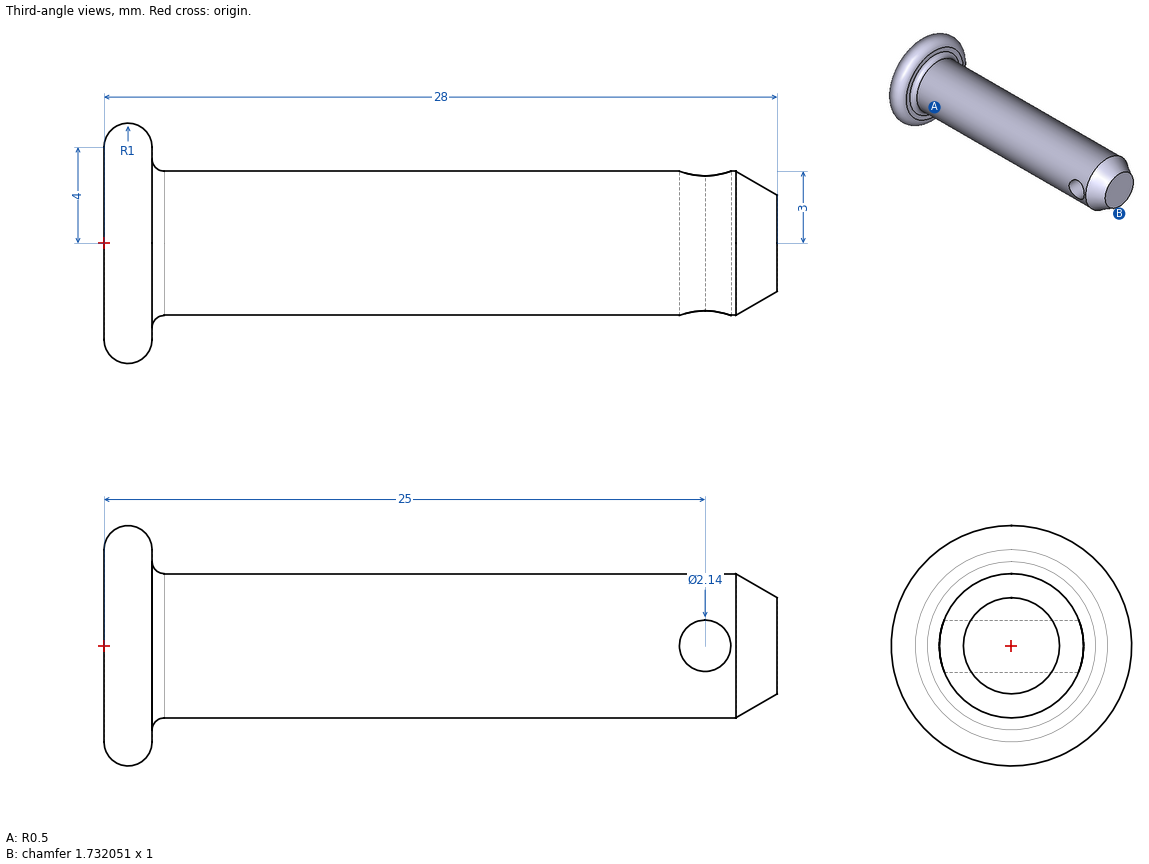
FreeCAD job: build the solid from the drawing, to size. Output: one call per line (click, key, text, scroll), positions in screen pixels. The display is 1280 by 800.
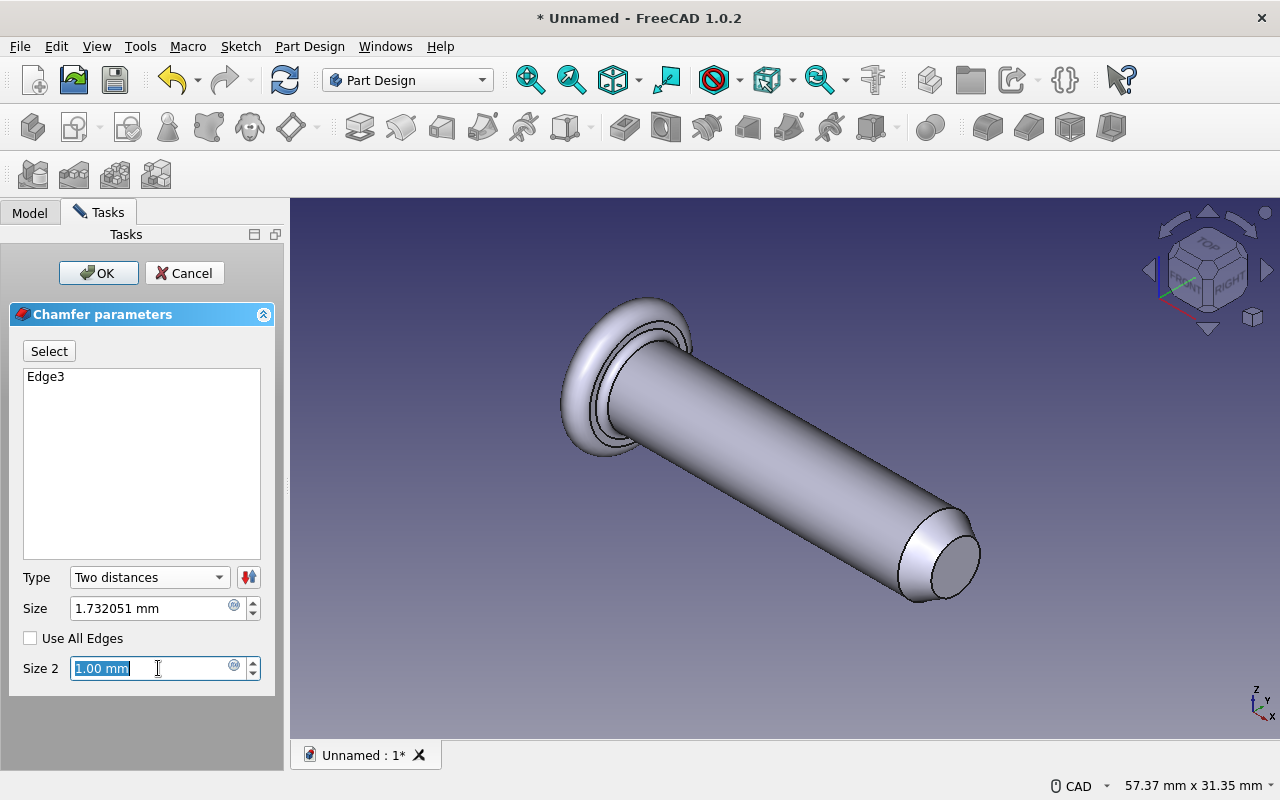
text(1)
key(Tab)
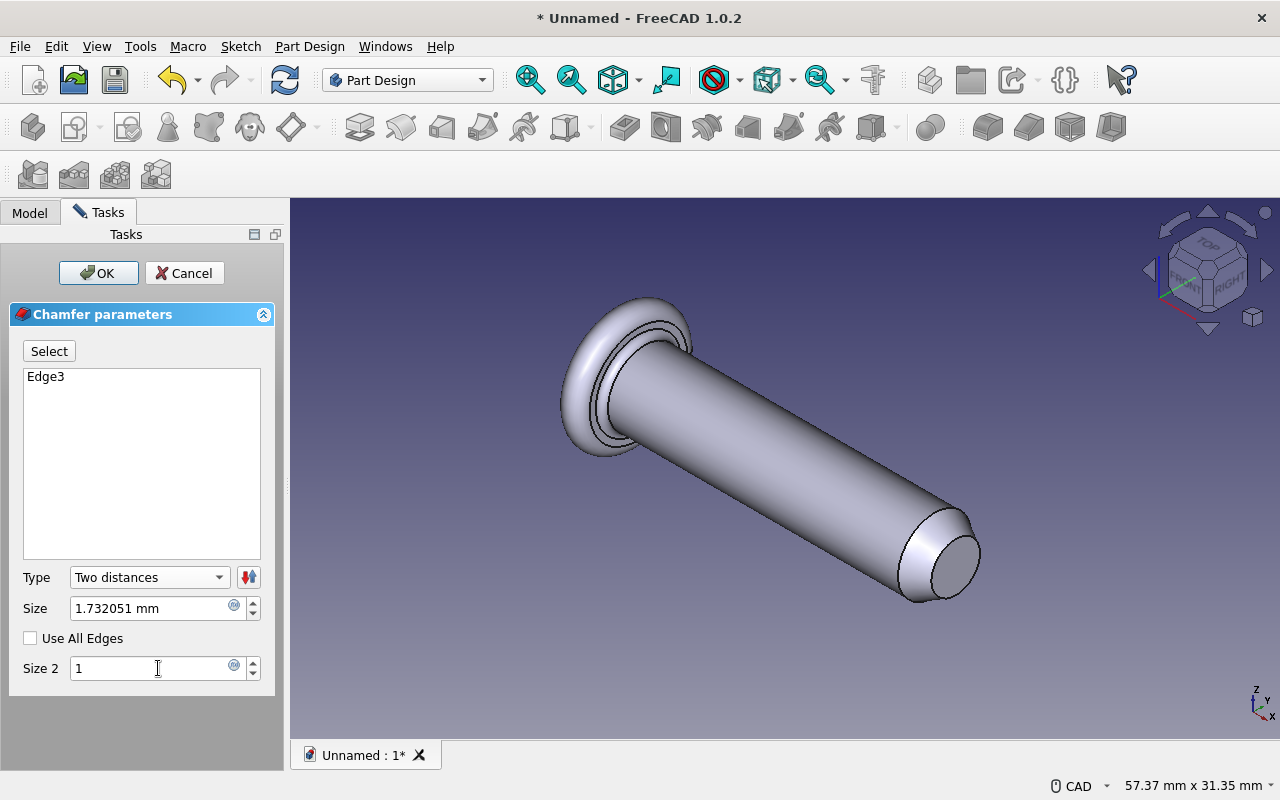
click(99, 273)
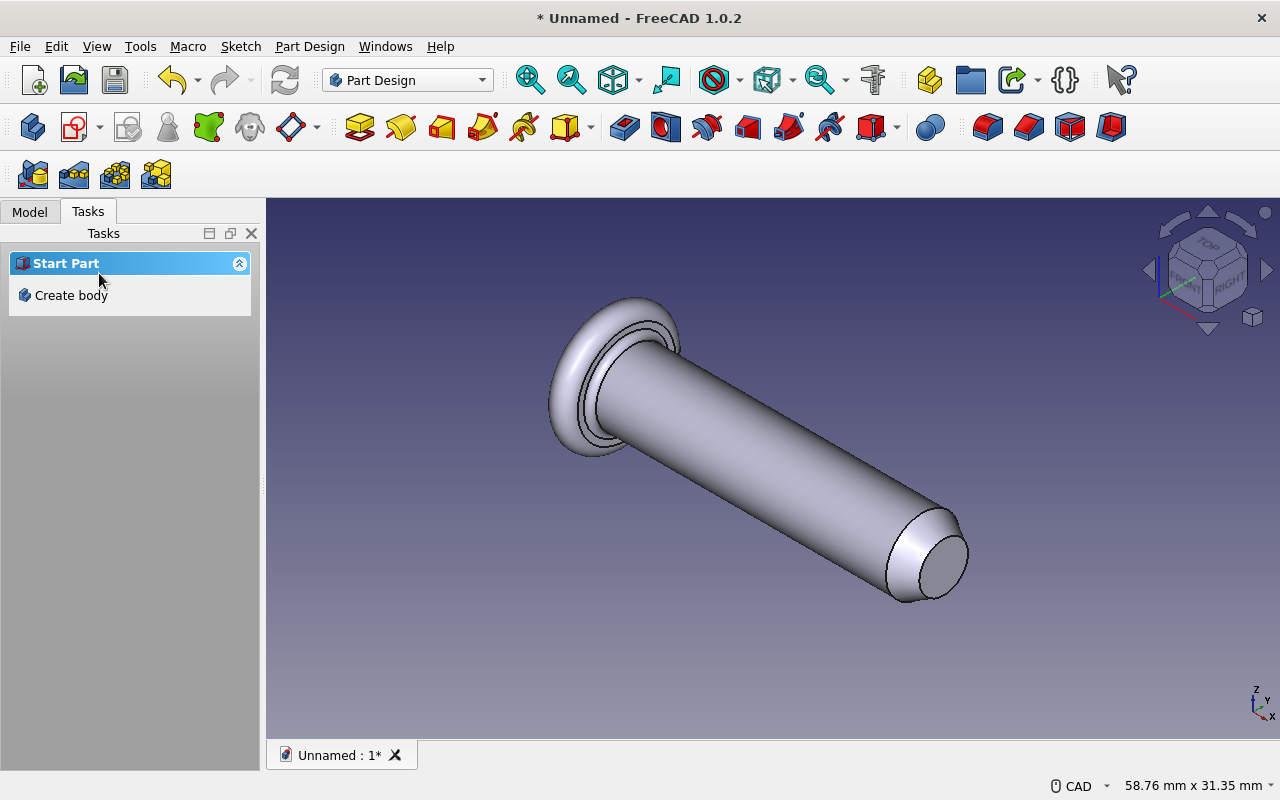
click(74, 128)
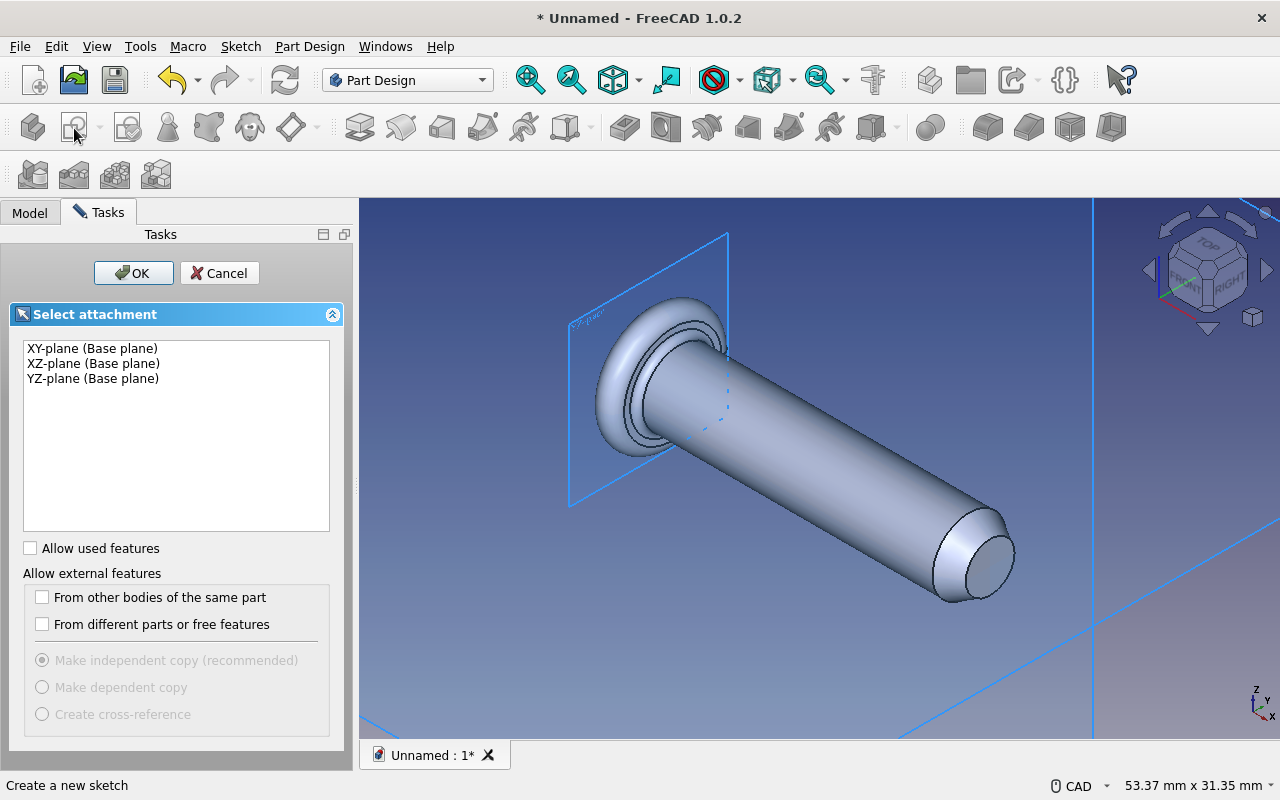
click(84, 364)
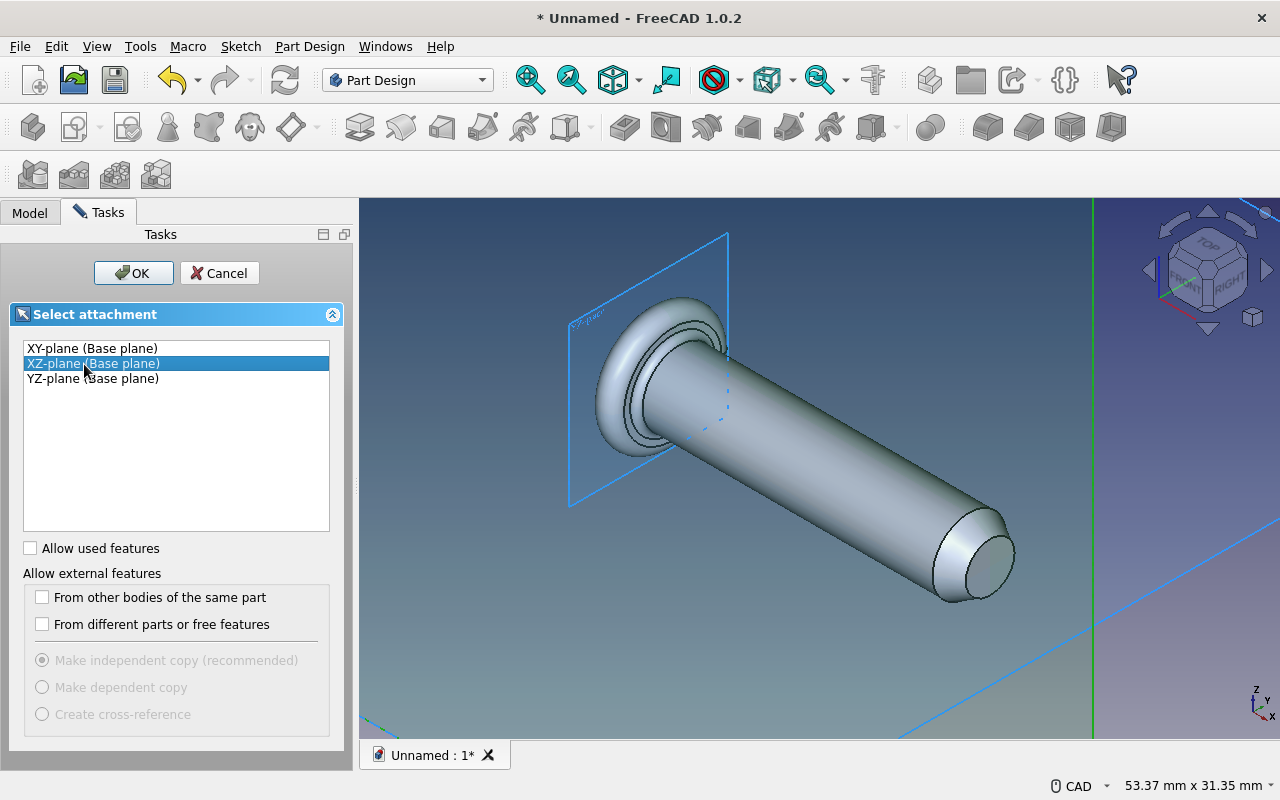
click(134, 273)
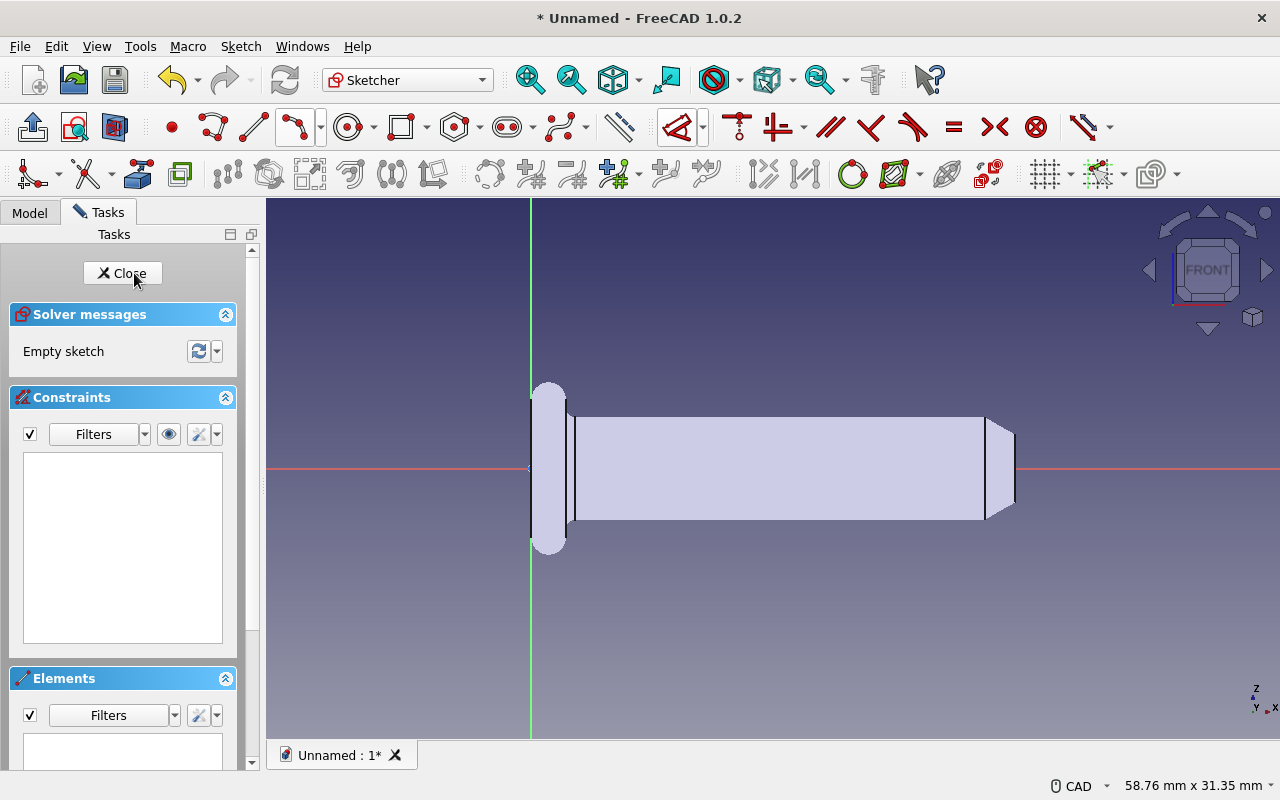
click(115, 128)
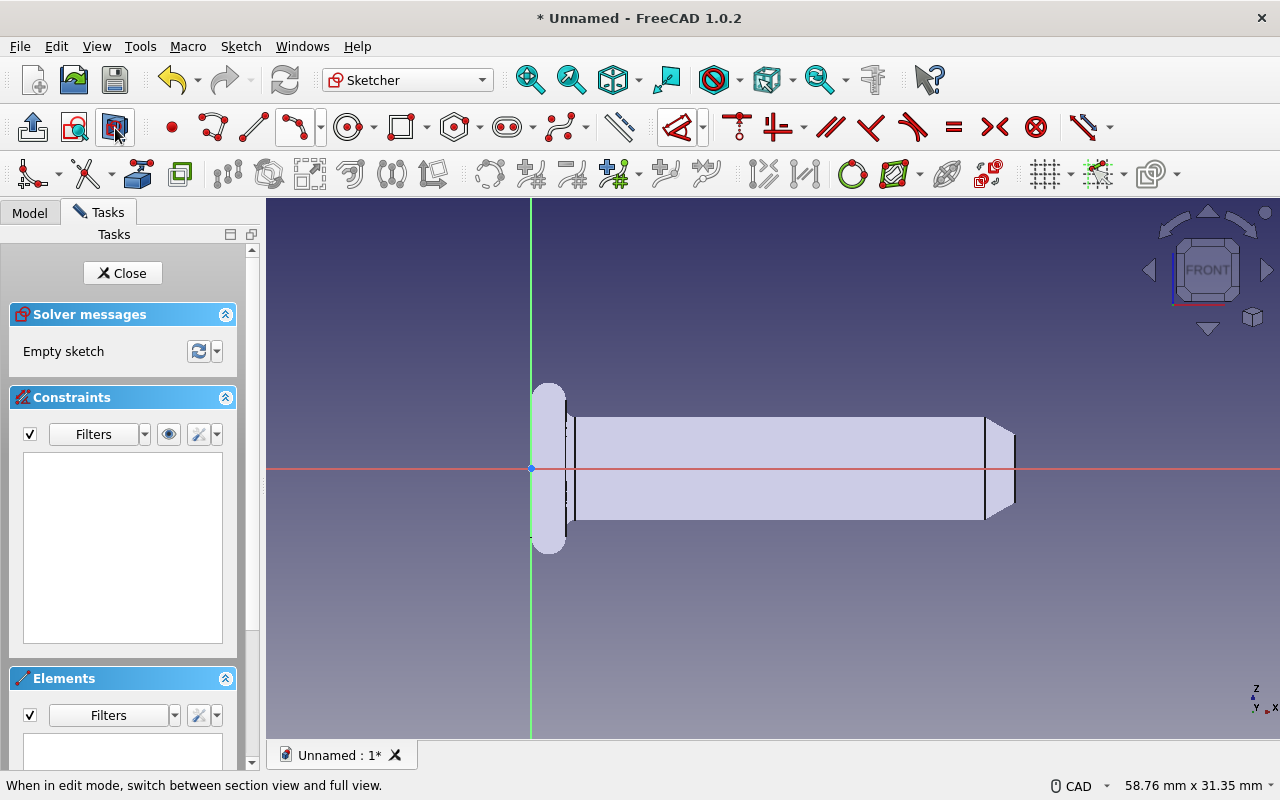
scroll(995, 469, up, 11)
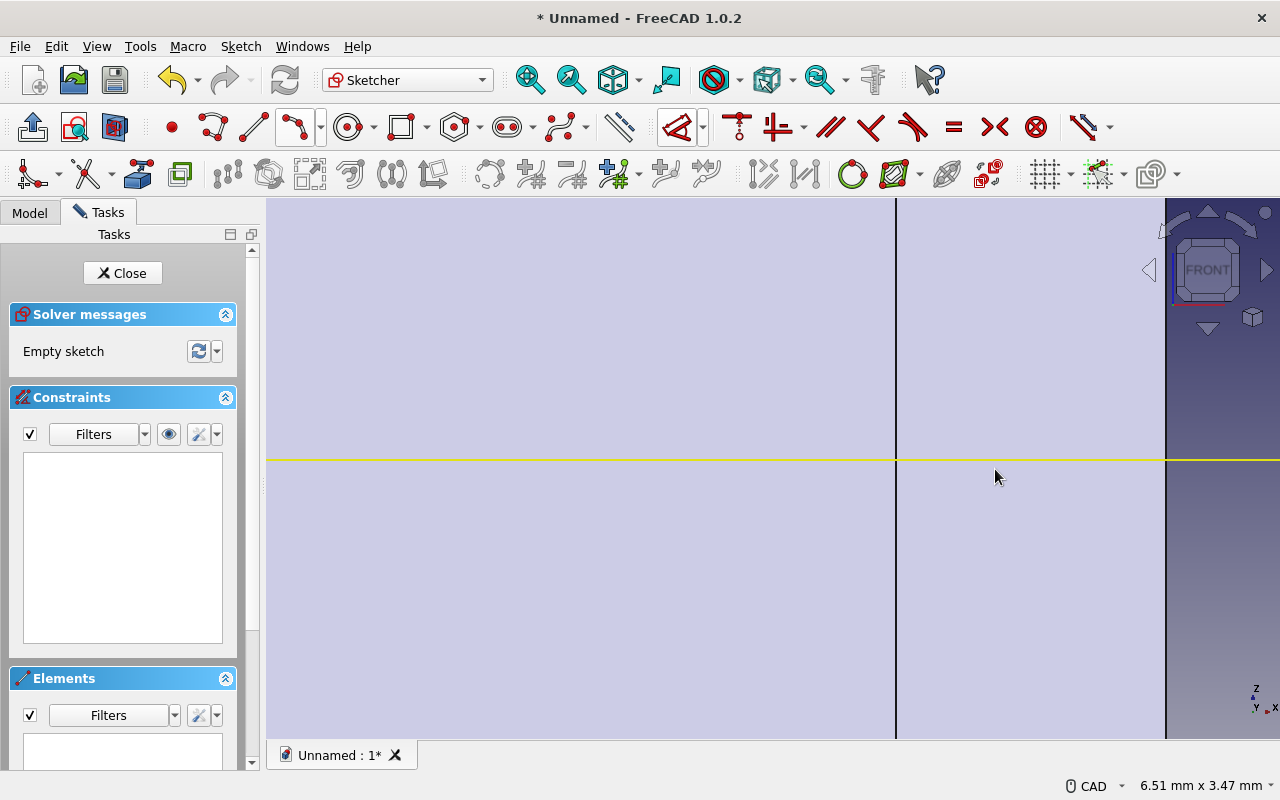
click(348, 128)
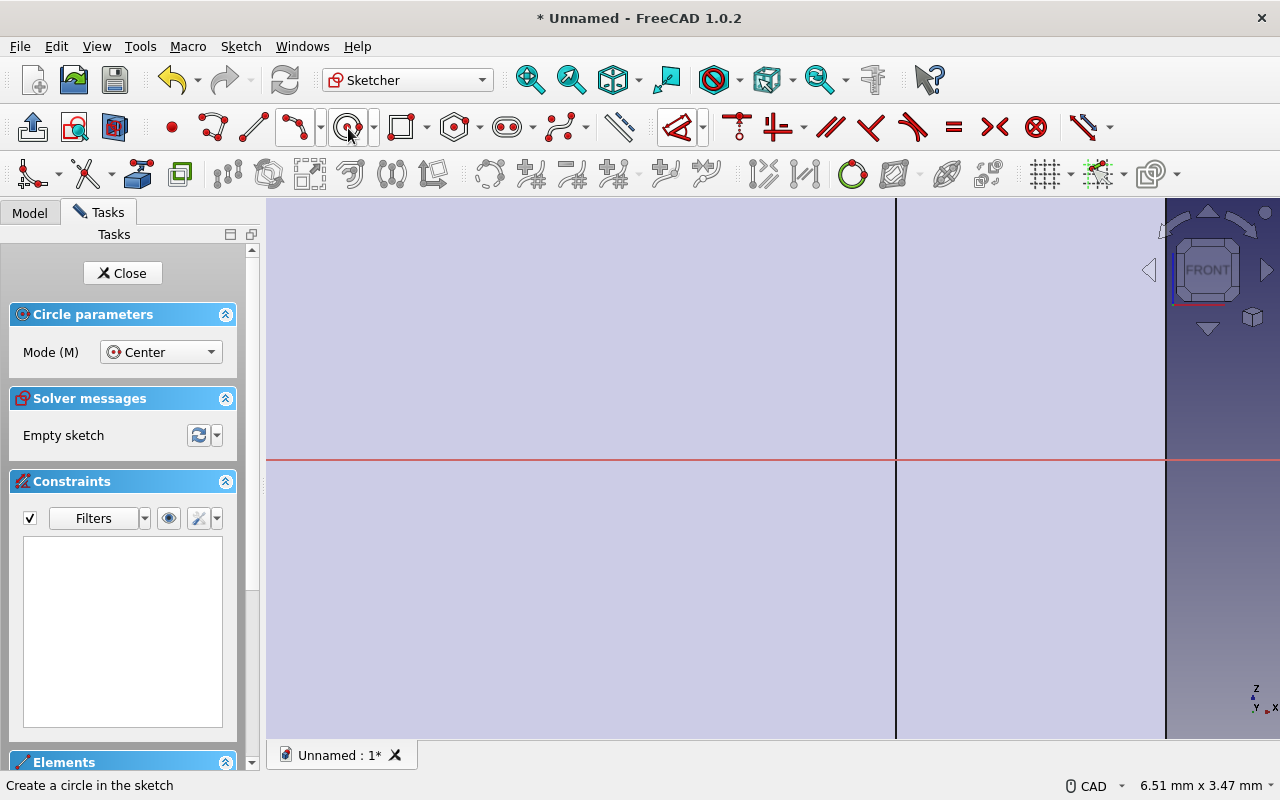
click(699, 460)
click(817, 343)
key(Escape)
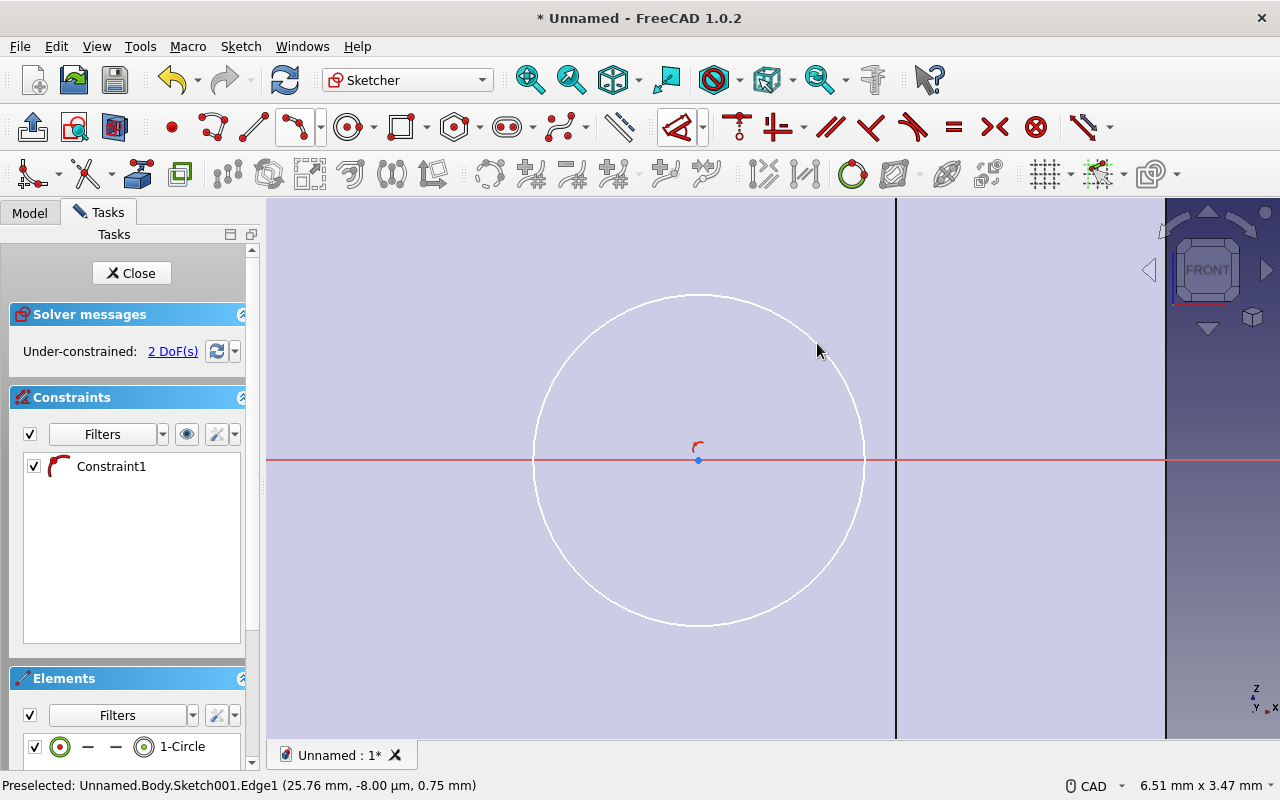
click(816, 343)